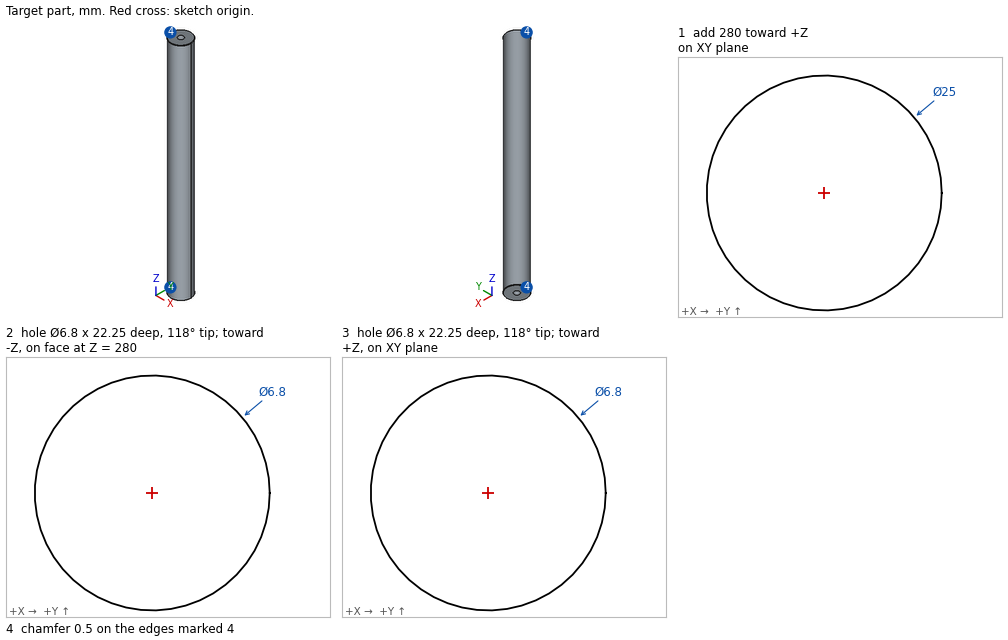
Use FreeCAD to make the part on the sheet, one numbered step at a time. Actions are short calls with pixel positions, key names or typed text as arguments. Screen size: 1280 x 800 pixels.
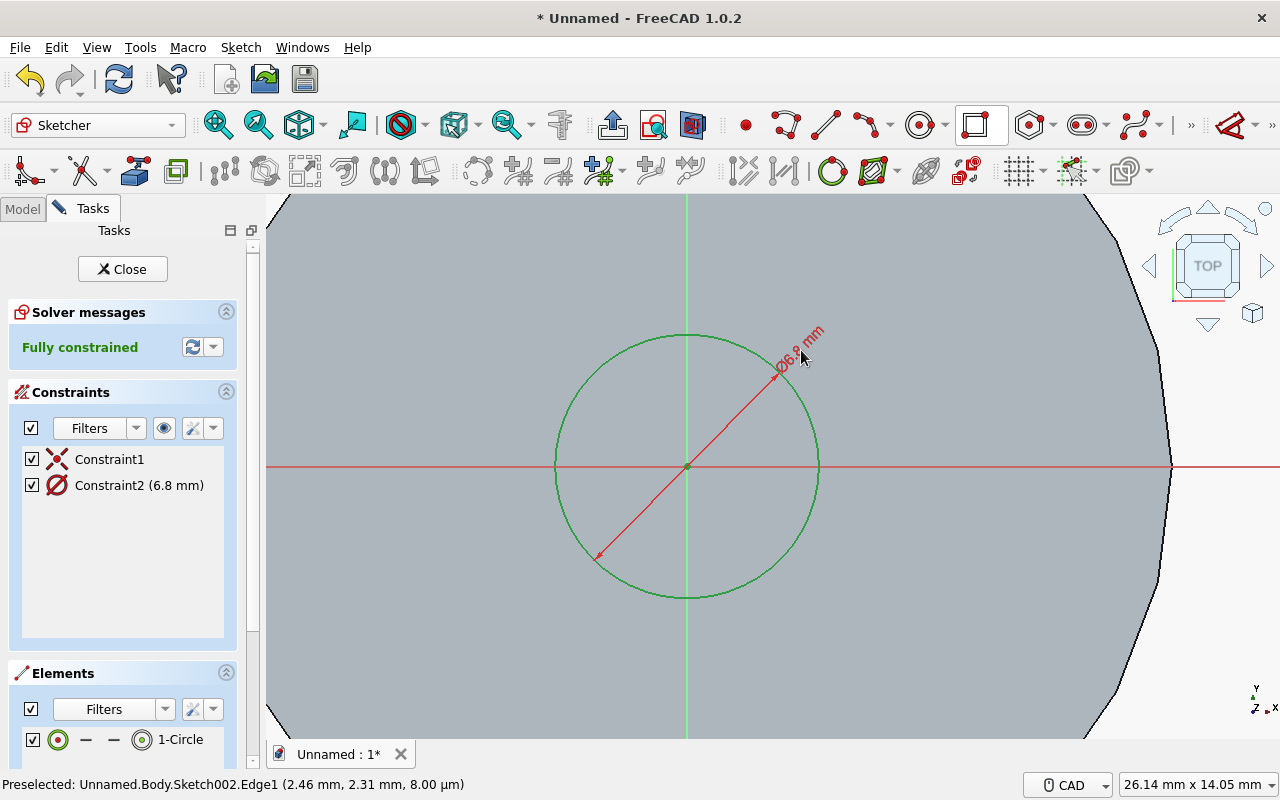
click(123, 269)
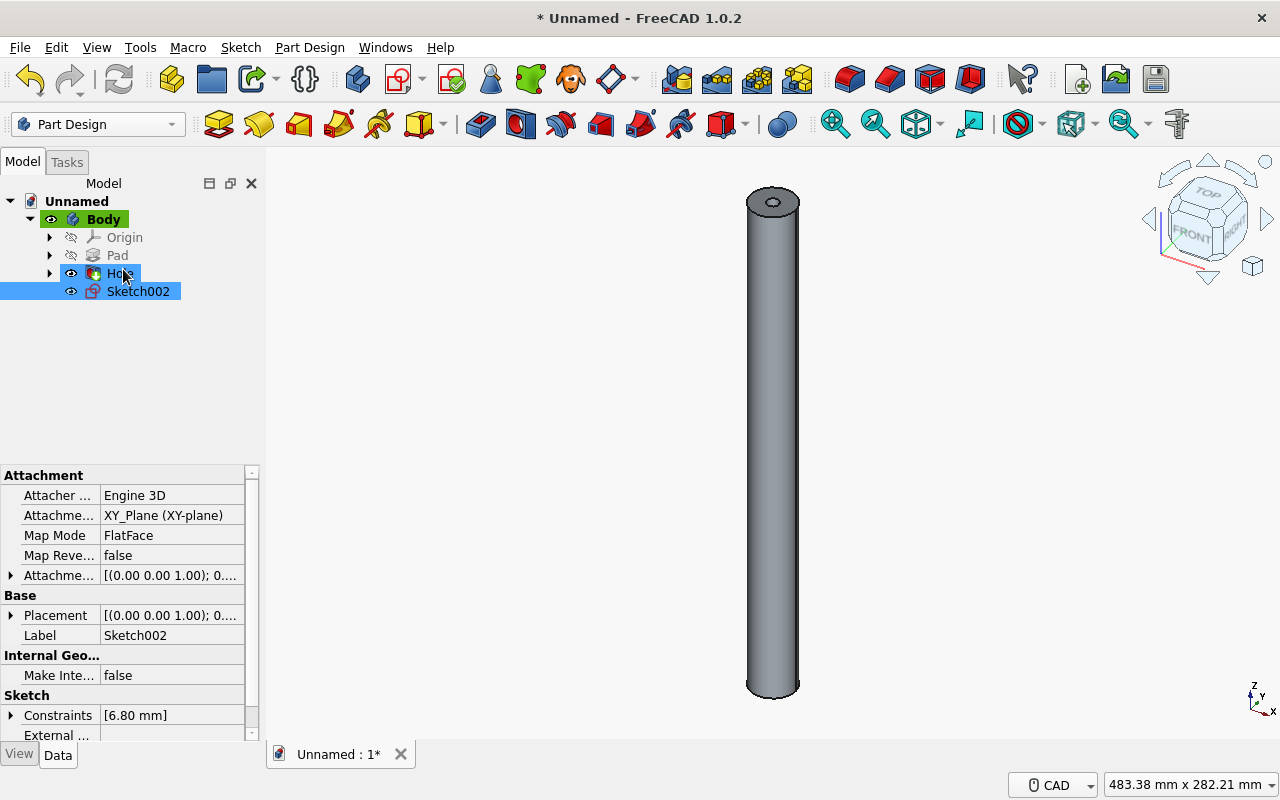
click(522, 124)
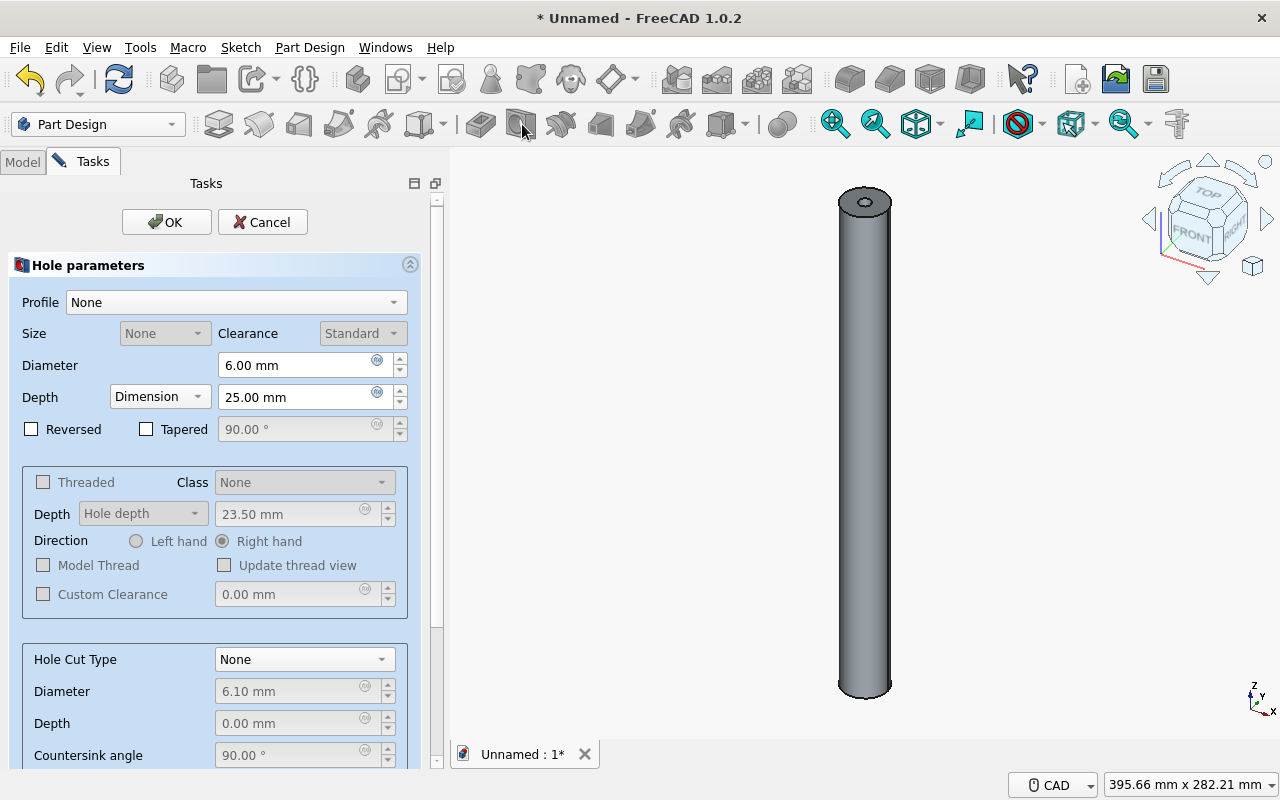
triple_click(305, 365)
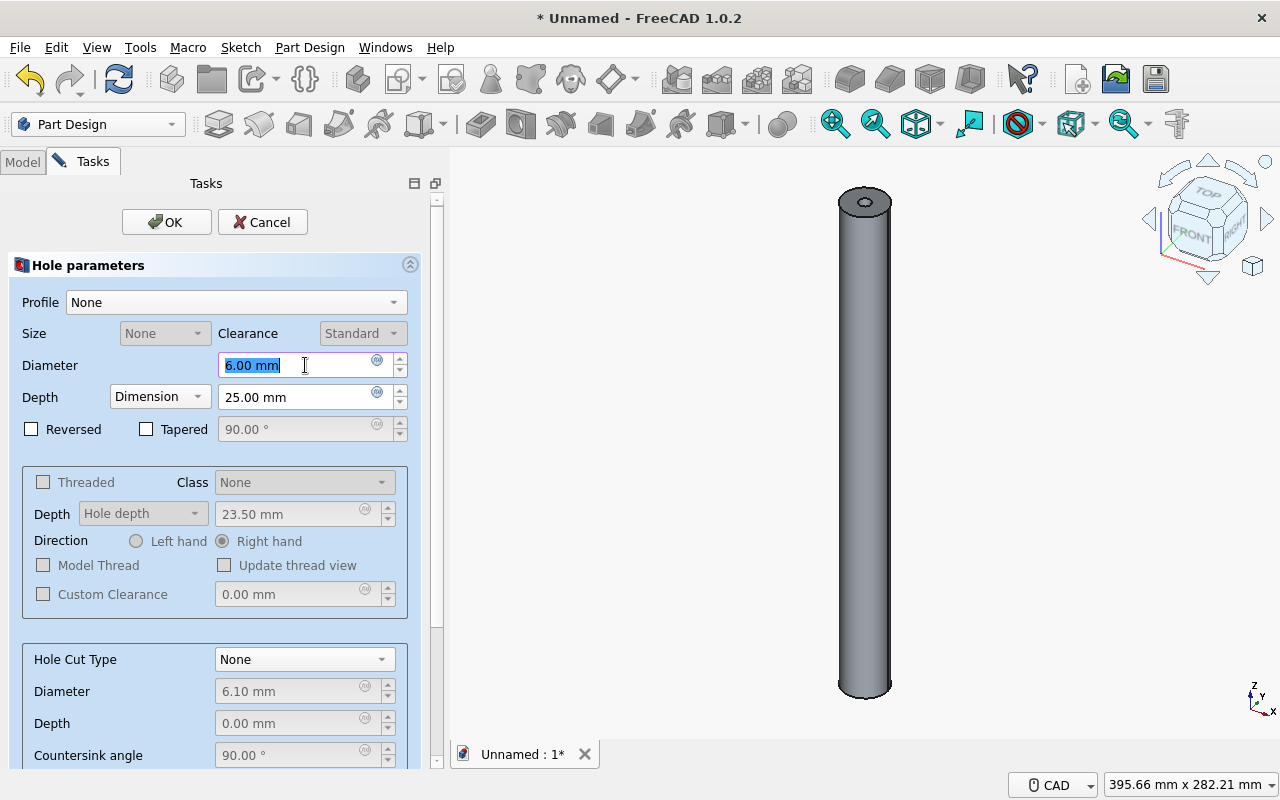
text(6.8)
key(Tab)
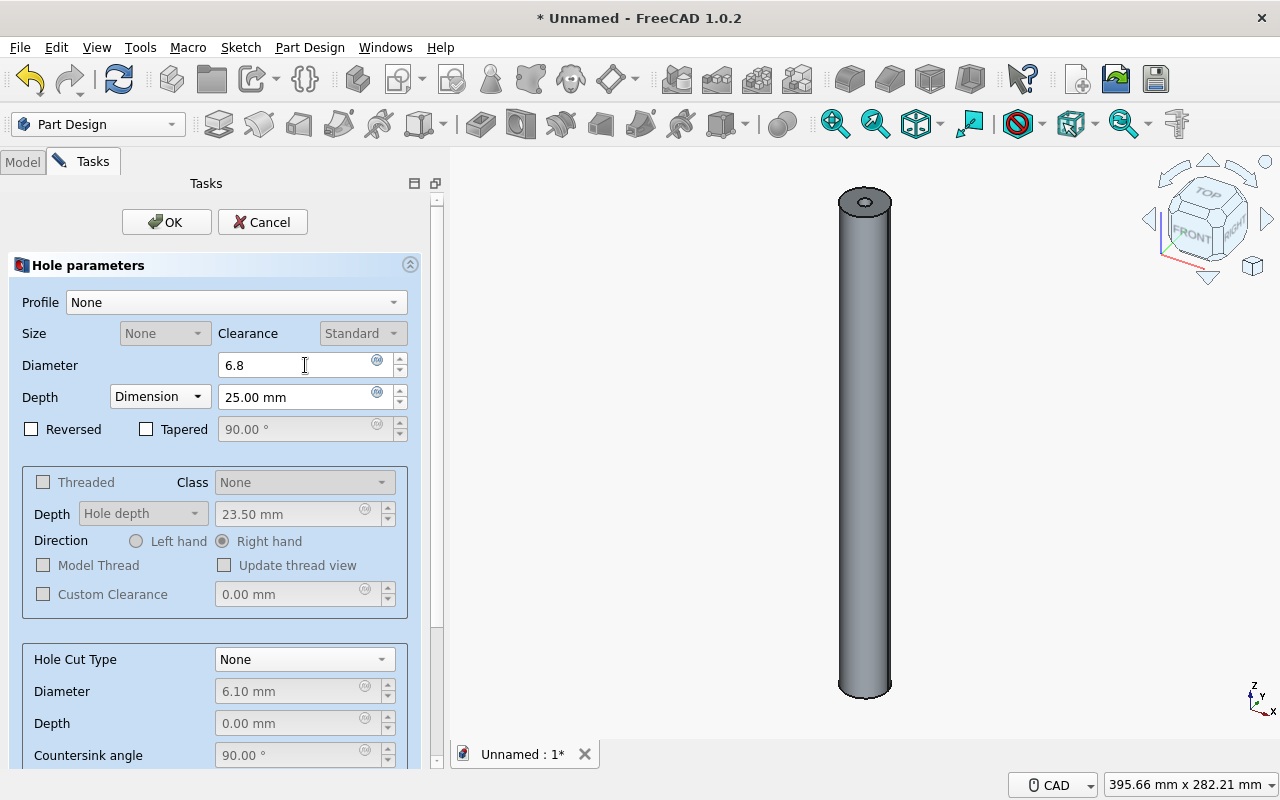
triple_click(305, 397)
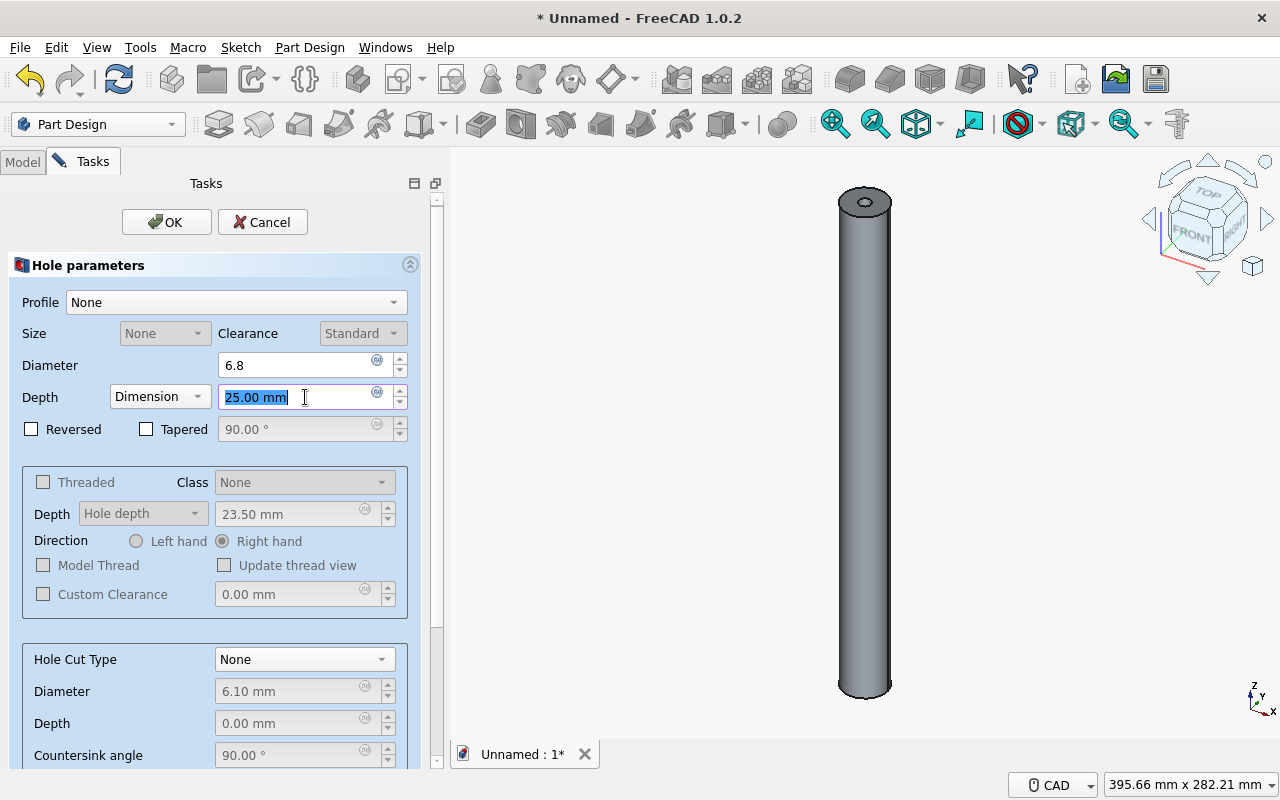
text(22.25)
key(Tab)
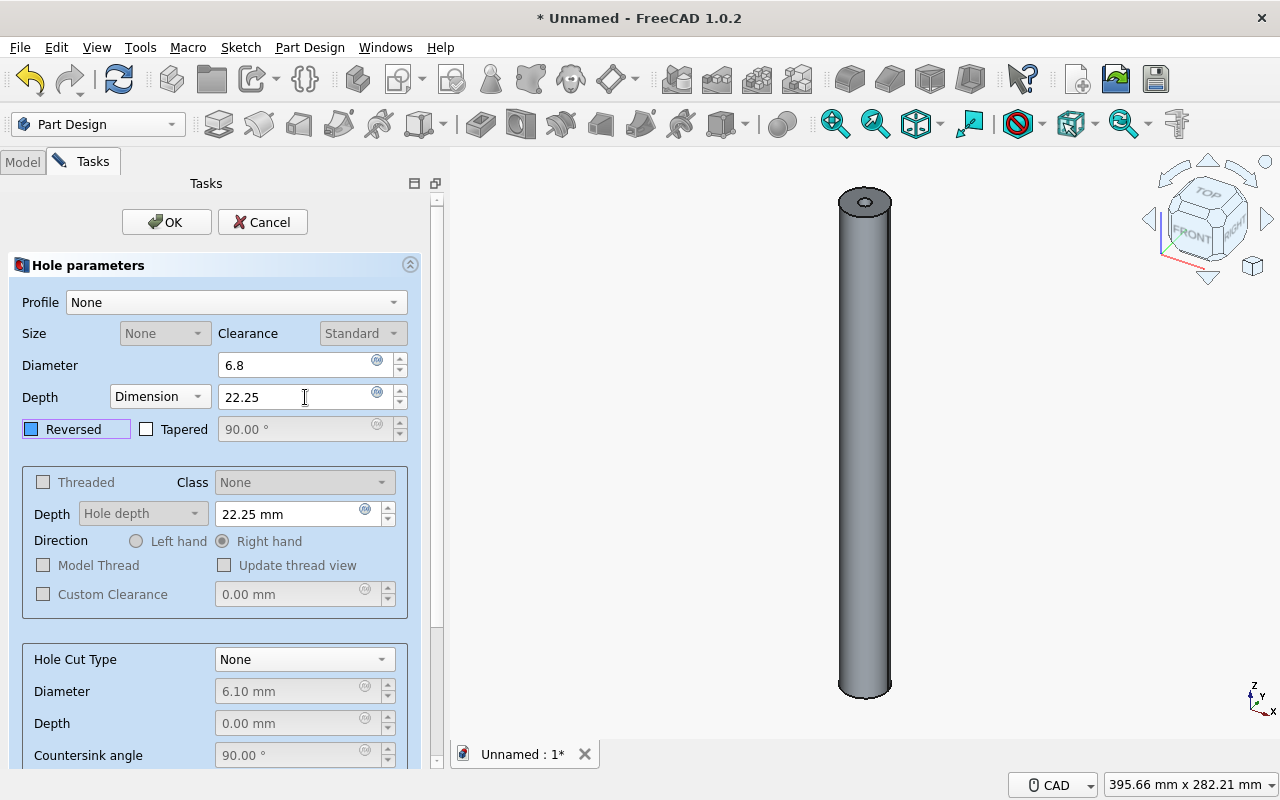
click(30, 429)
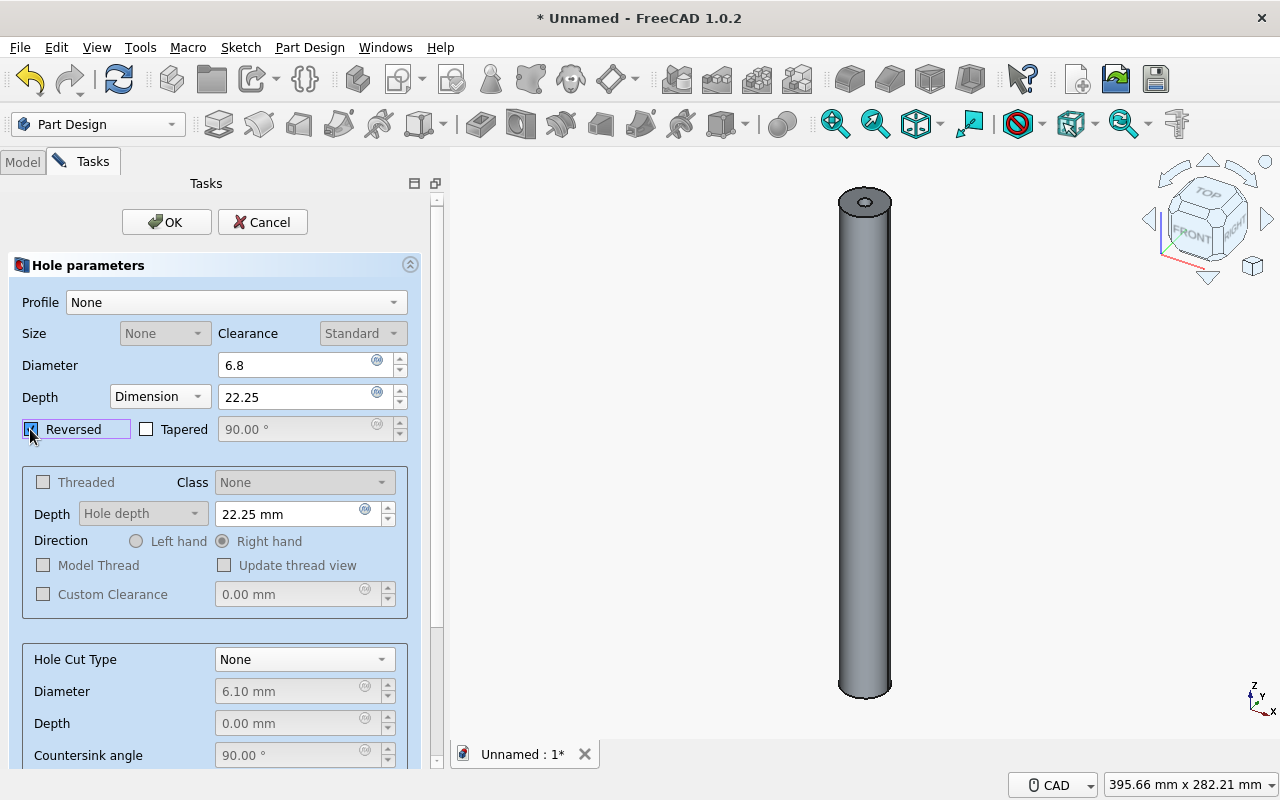
click(167, 222)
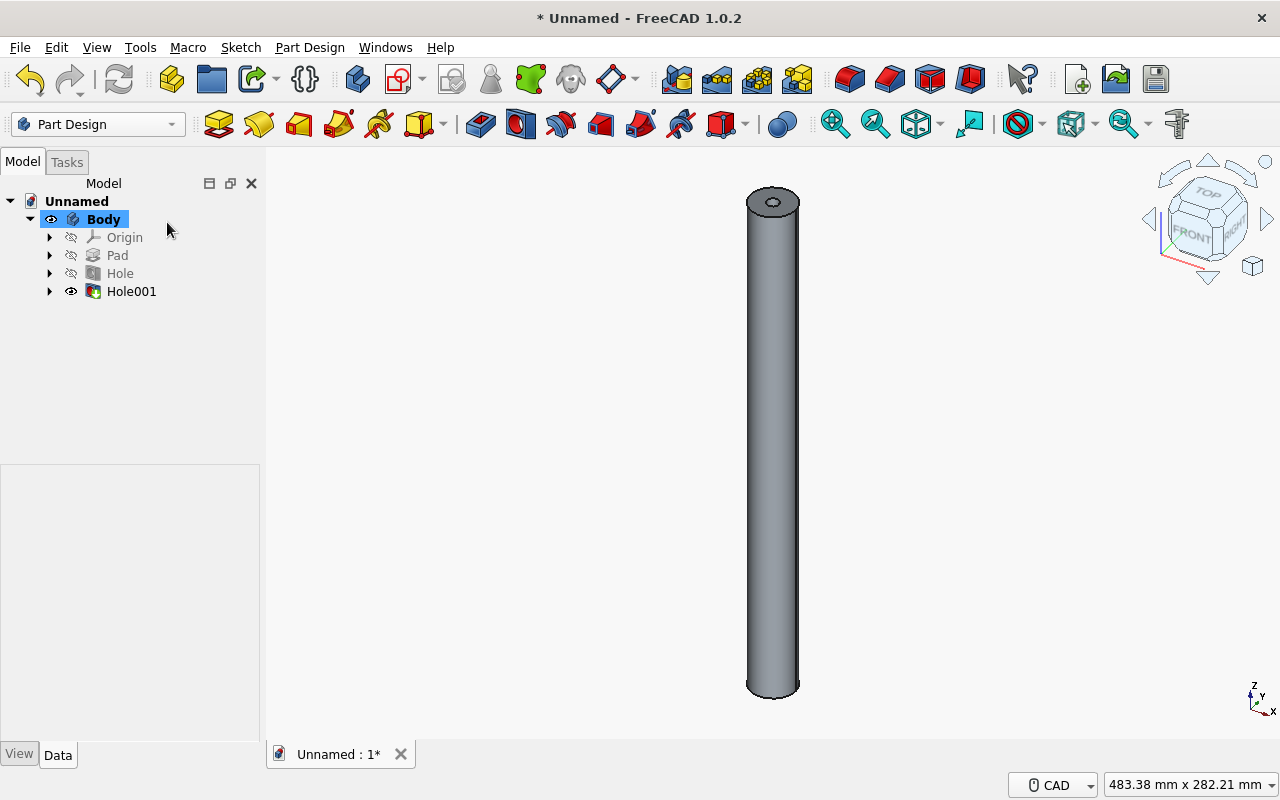
click(747, 203)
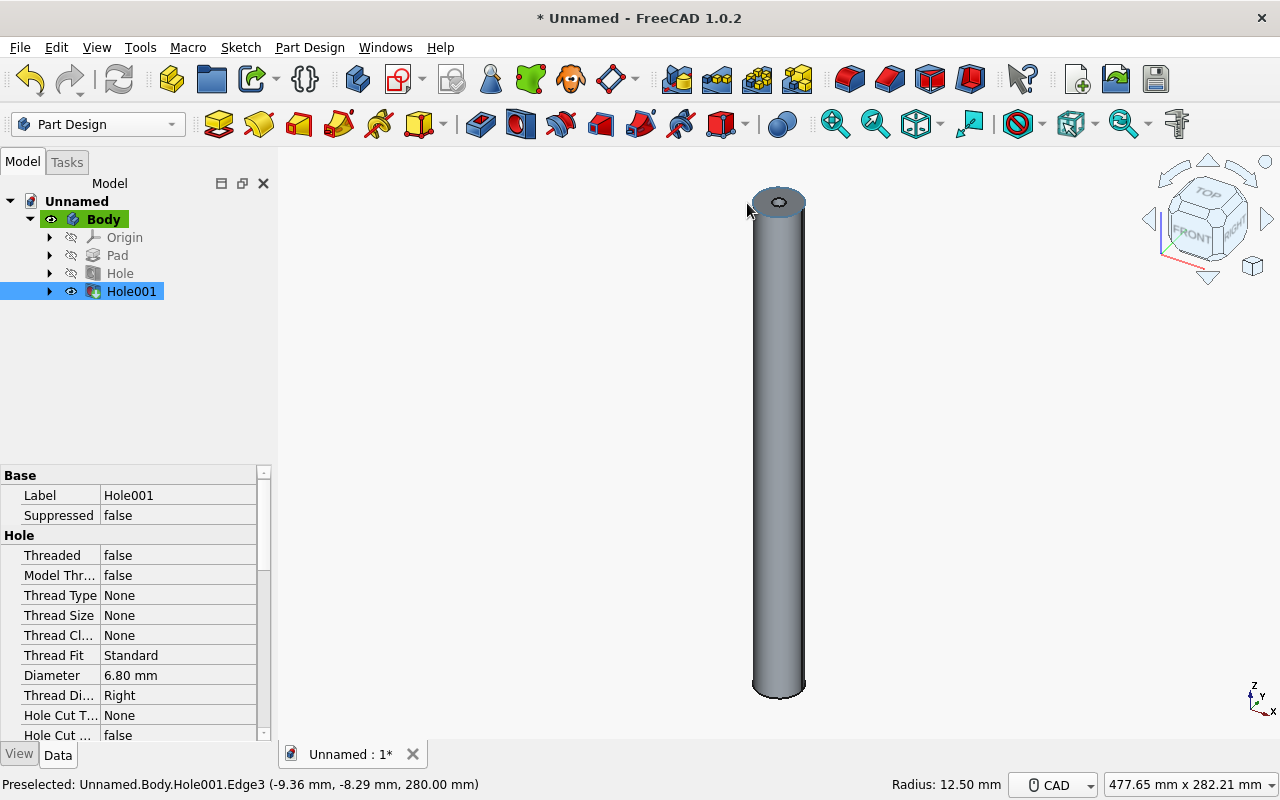
key(0)